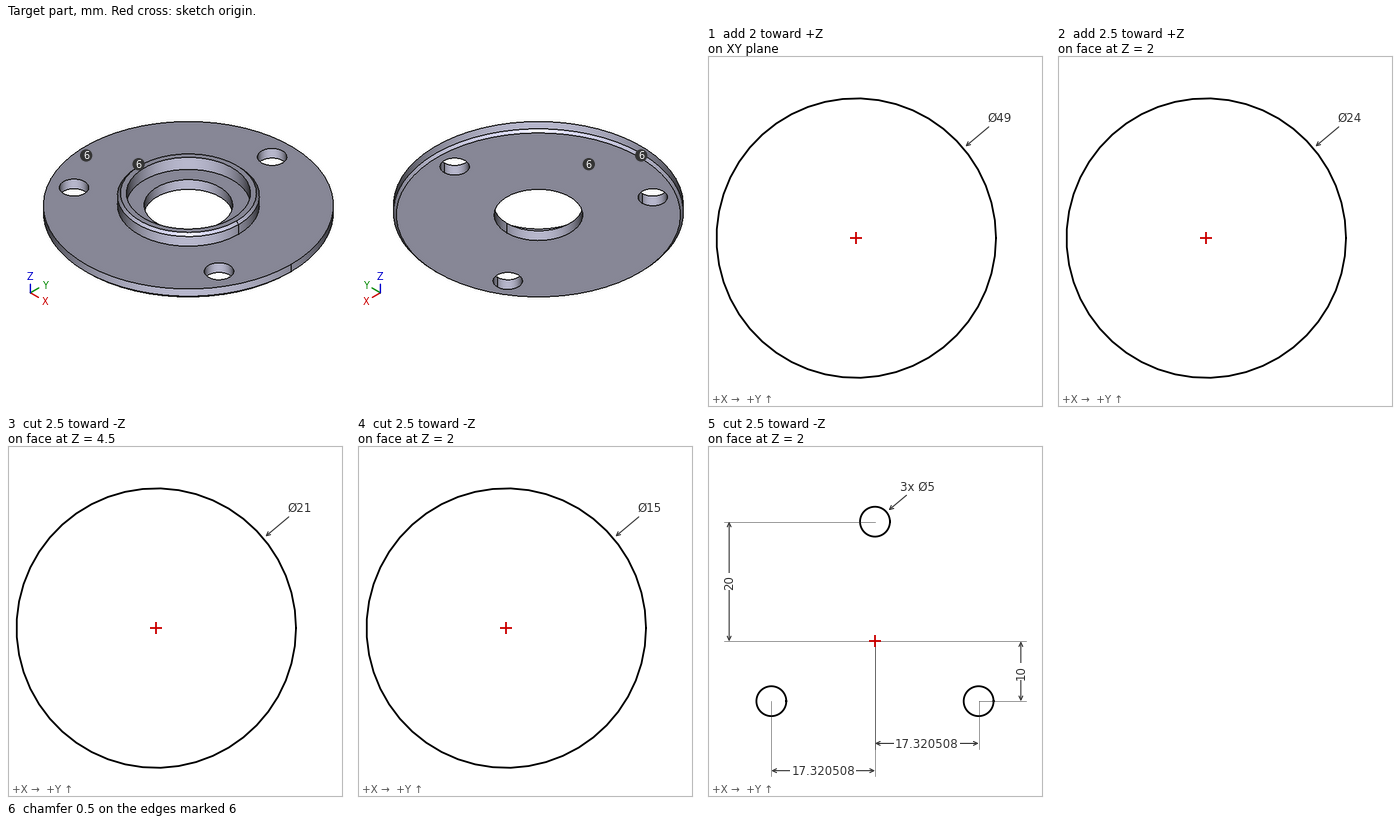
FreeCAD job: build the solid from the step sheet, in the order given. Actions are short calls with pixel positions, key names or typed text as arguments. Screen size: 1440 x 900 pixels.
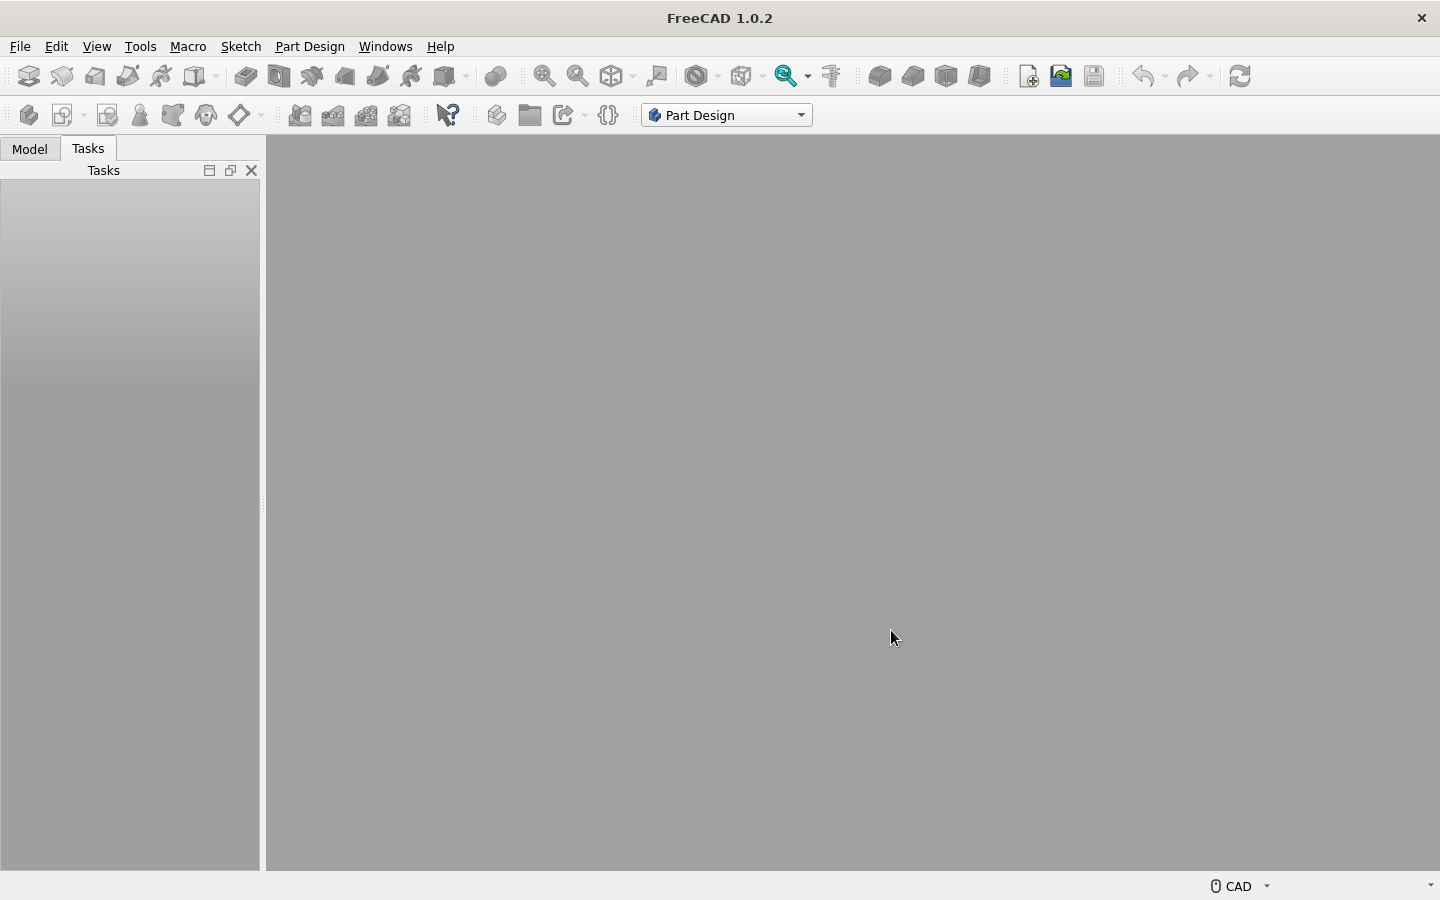
click(1028, 76)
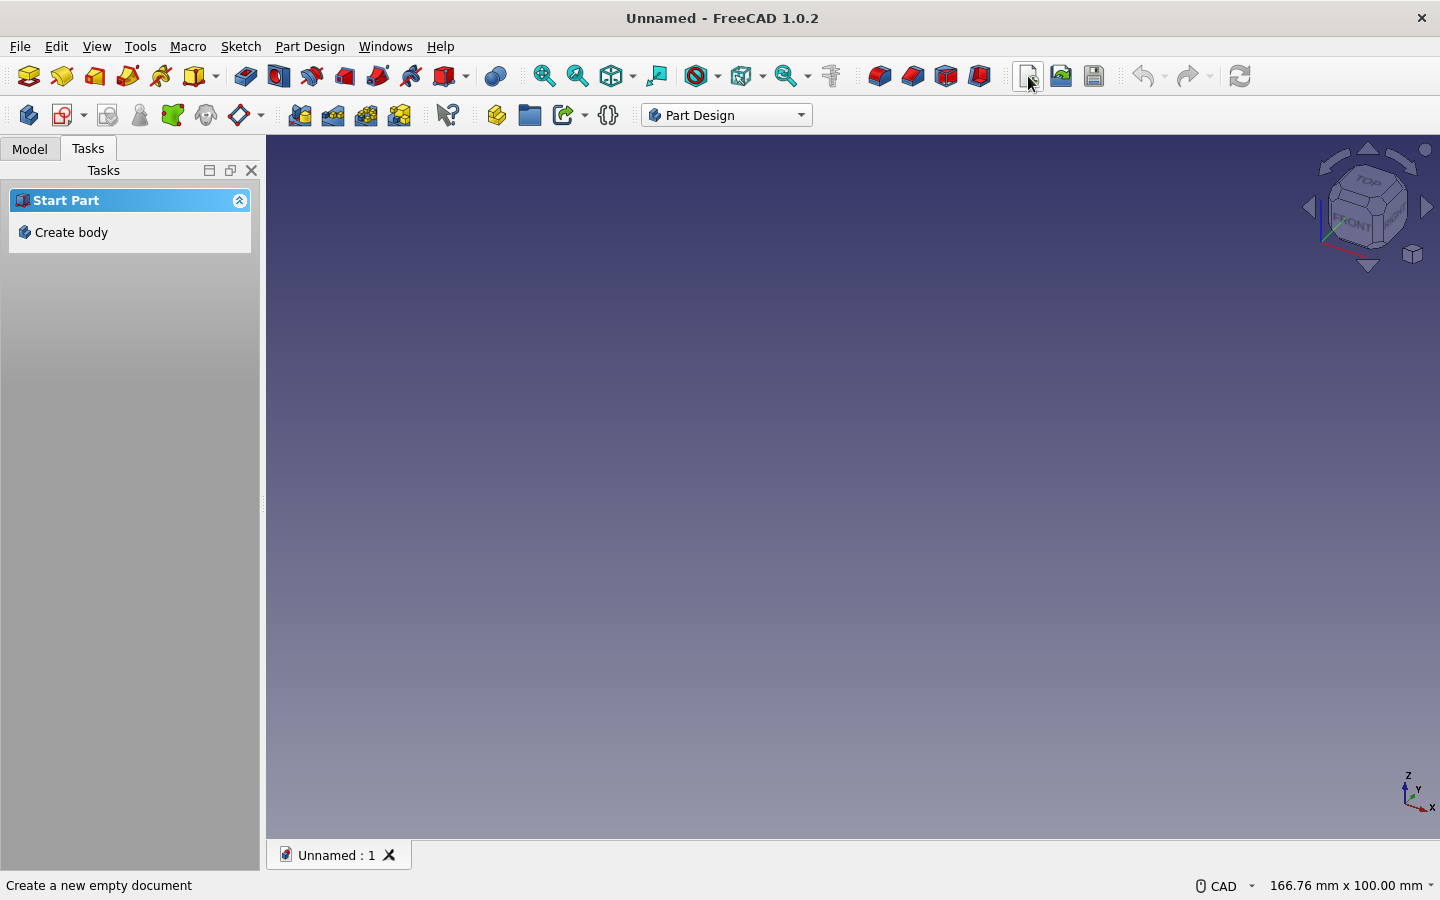
click(62, 116)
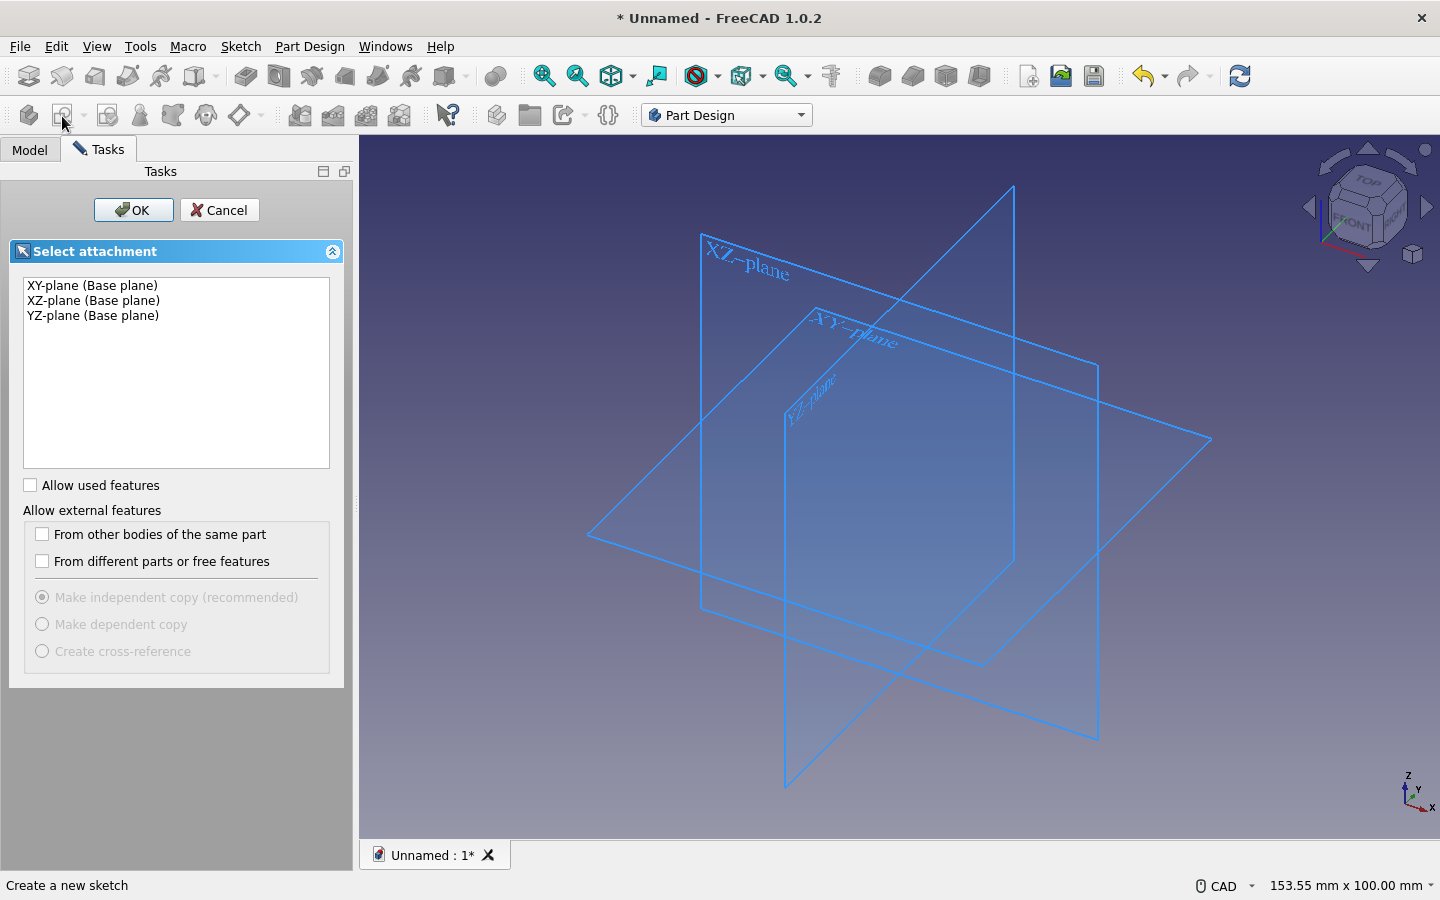
click(84, 286)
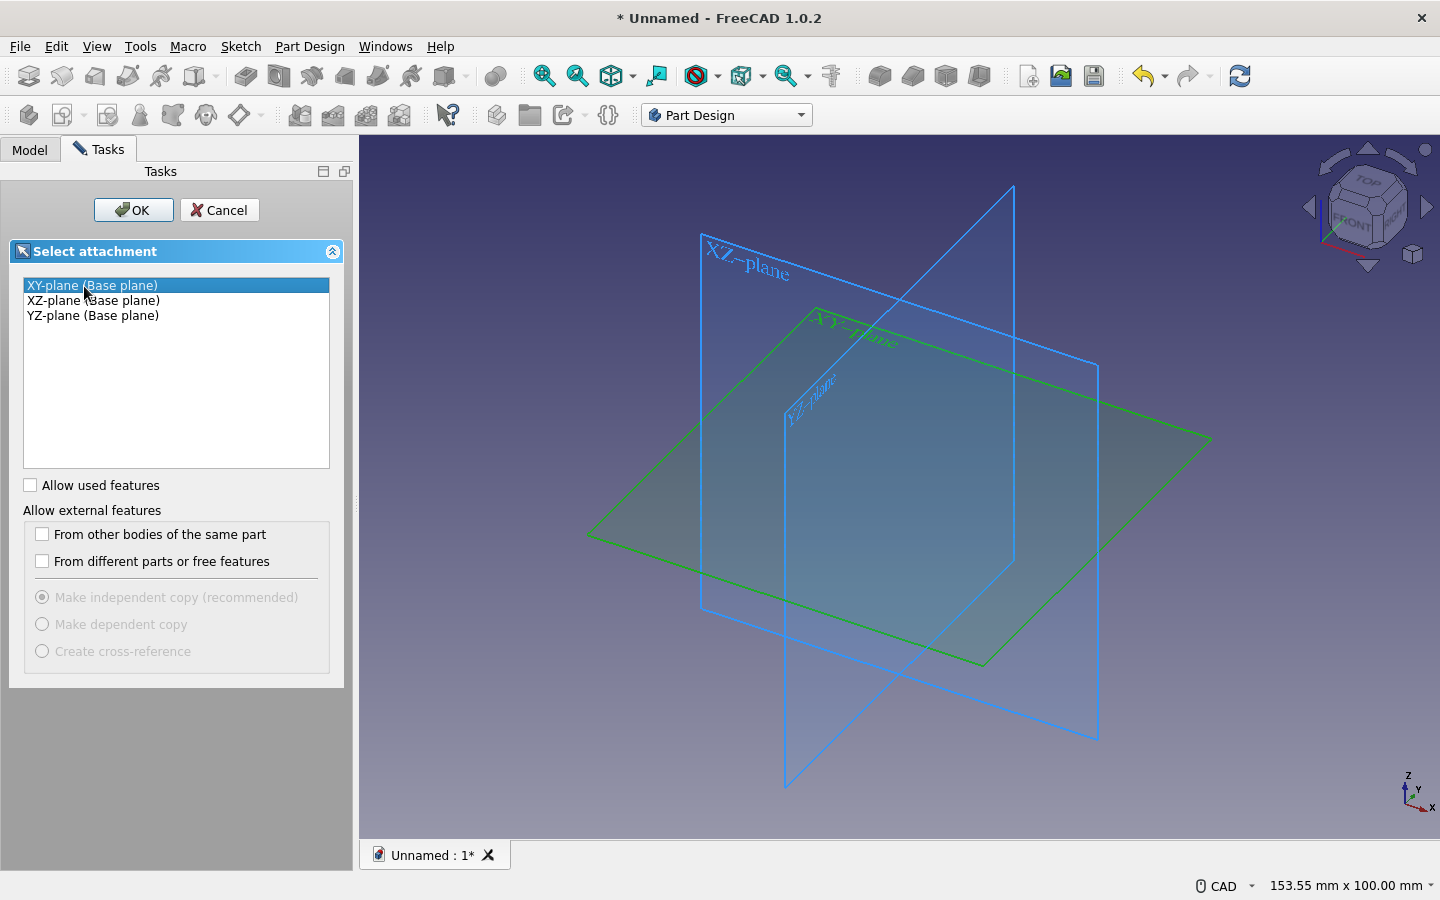
click(134, 210)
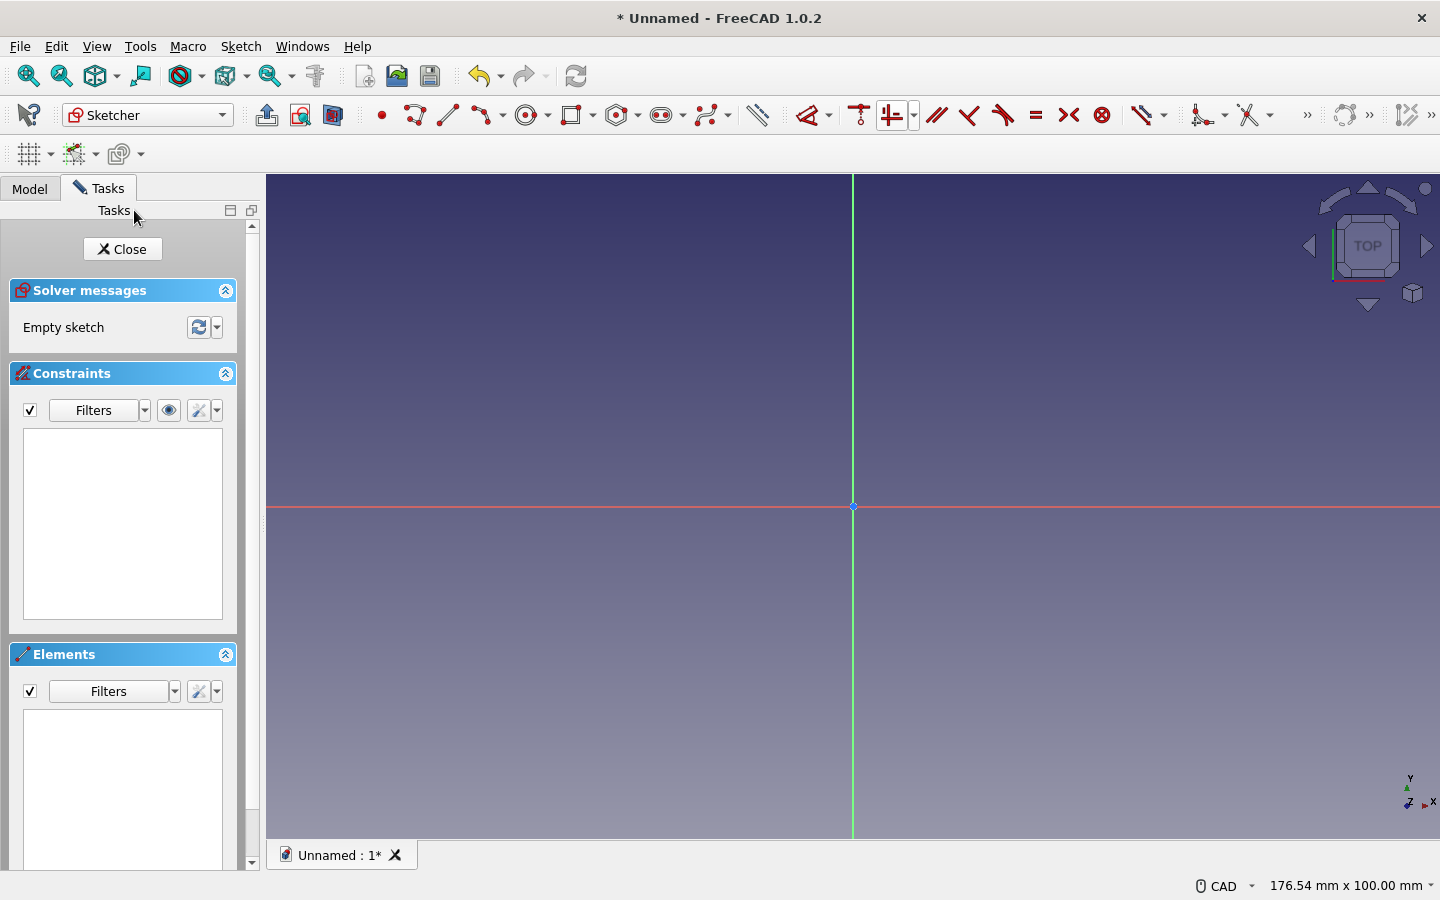
click(526, 116)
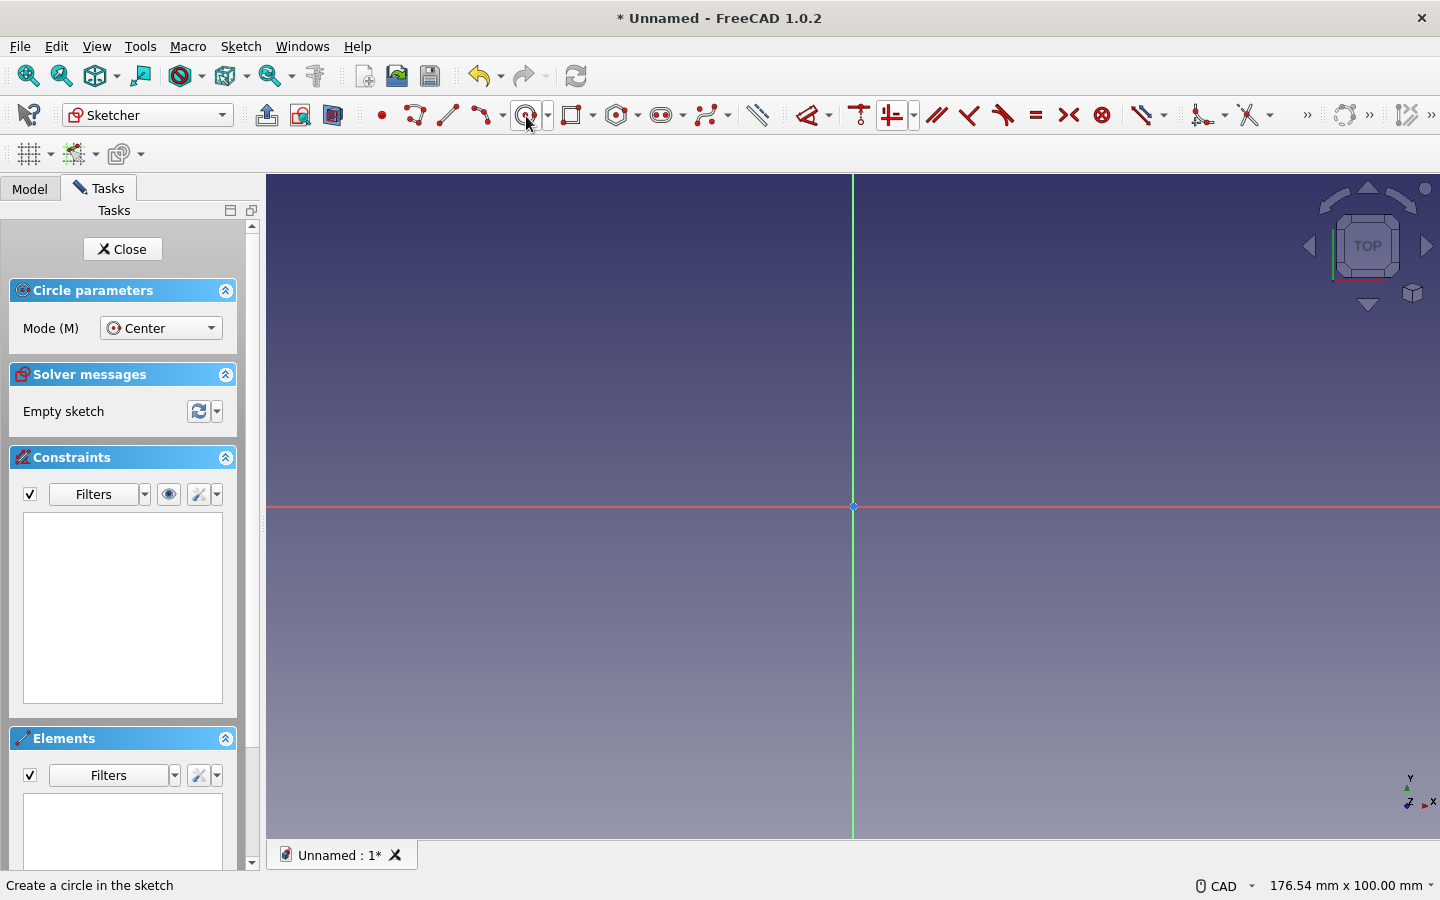
click(853, 506)
click(968, 391)
key(Escape)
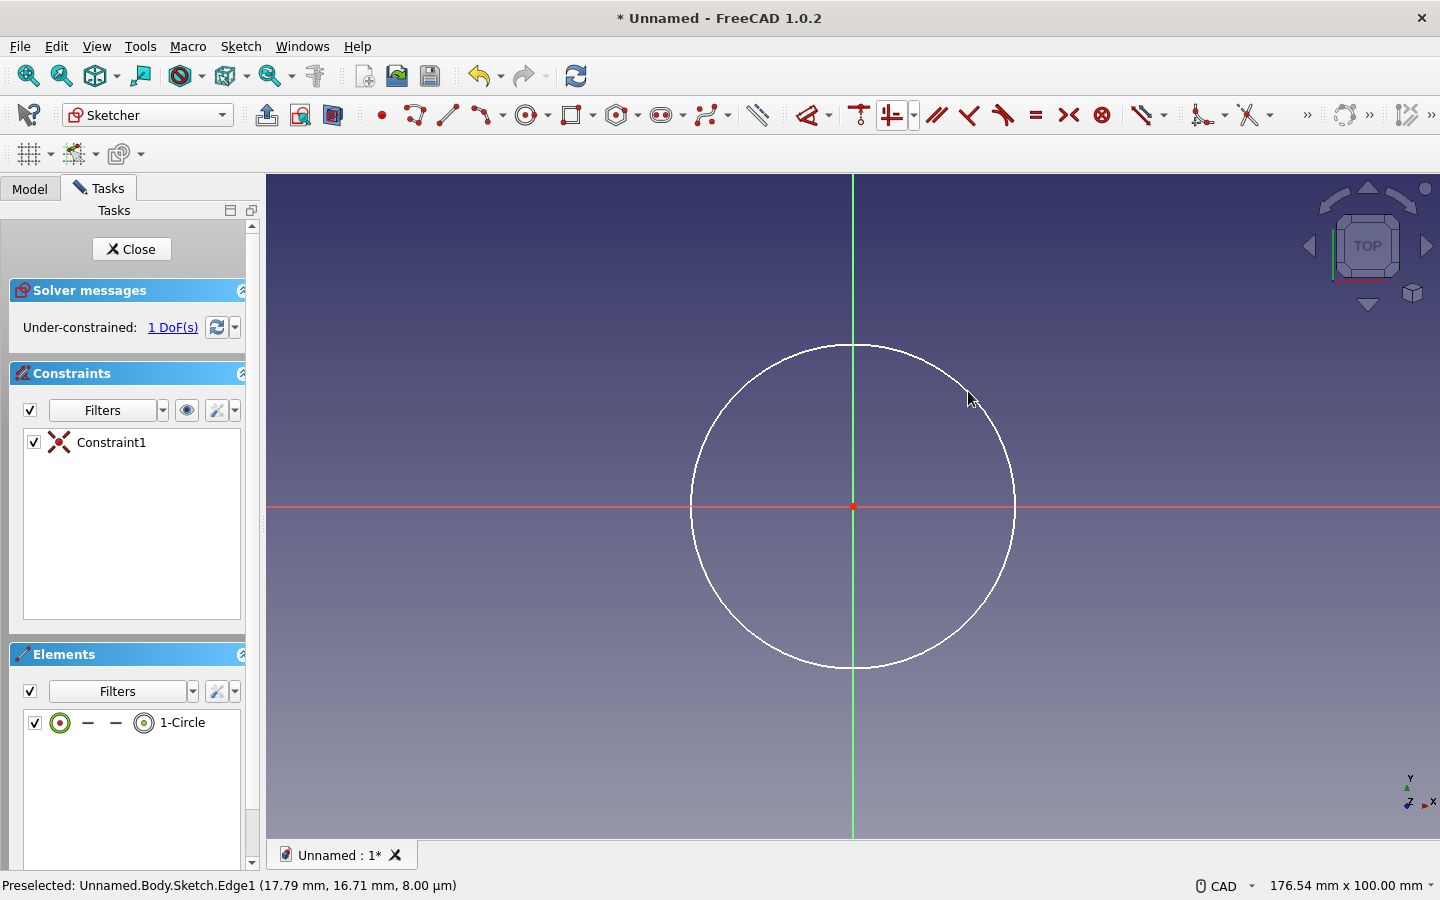
click(967, 391)